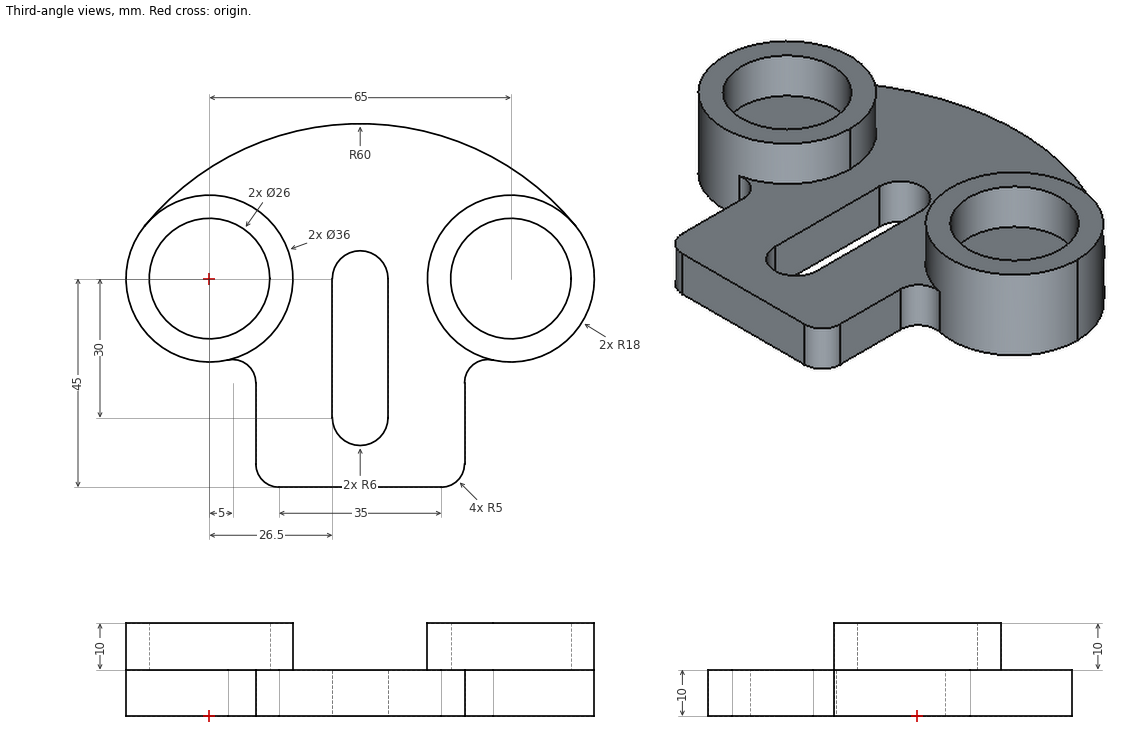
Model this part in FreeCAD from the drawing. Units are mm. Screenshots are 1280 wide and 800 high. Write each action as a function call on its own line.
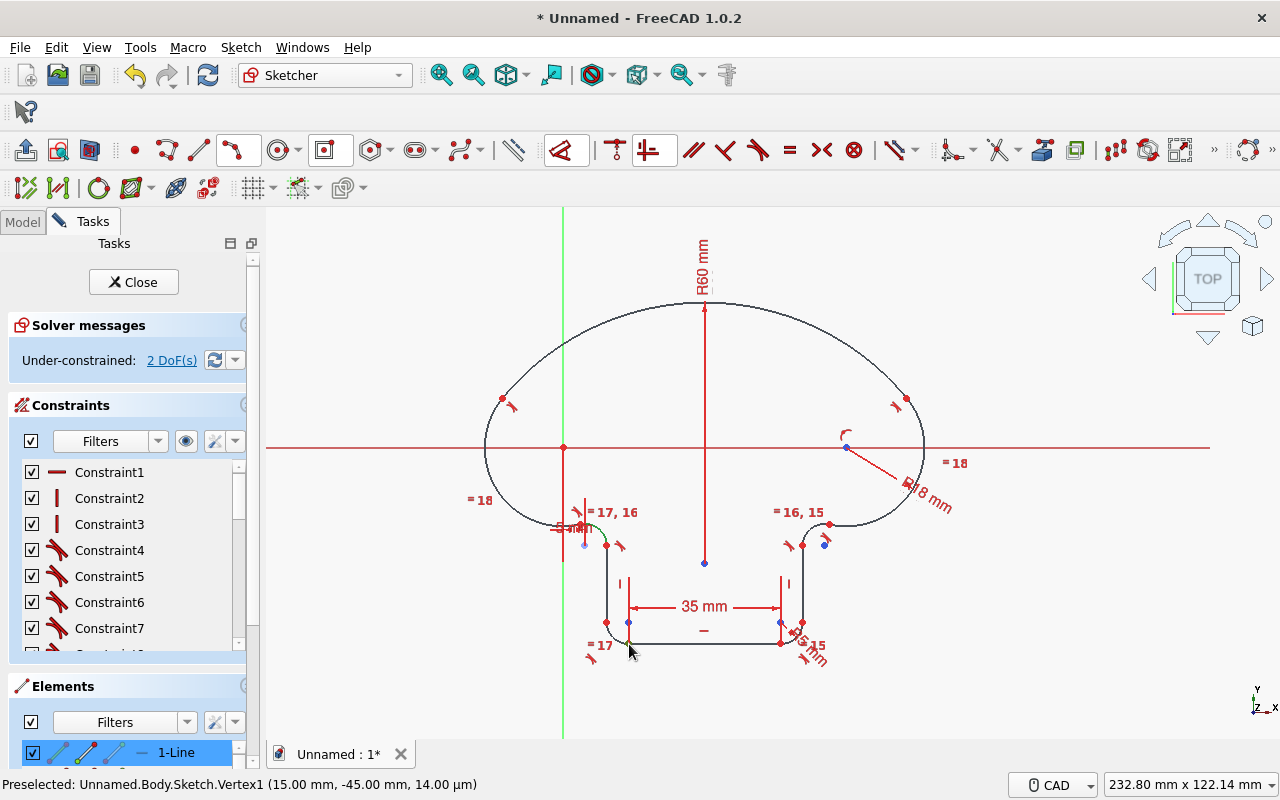
key(i)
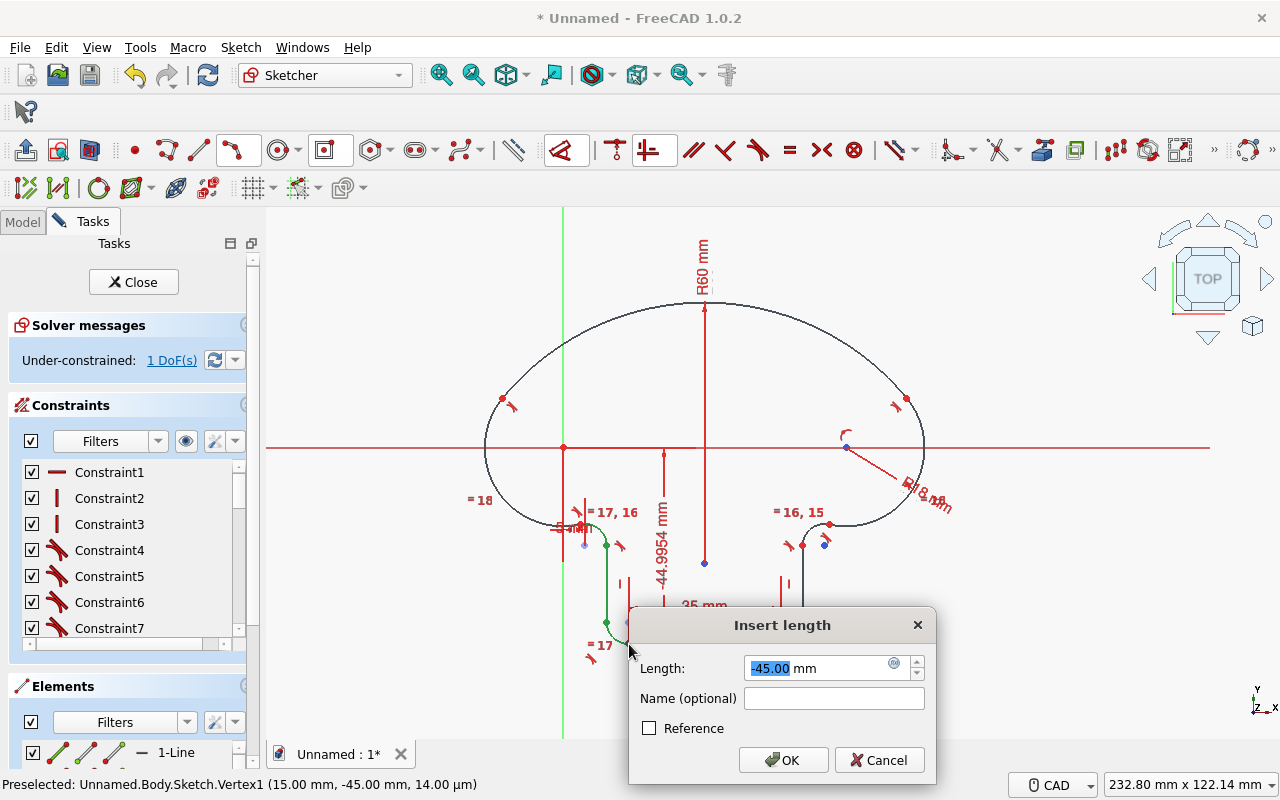
text(-45)
key(Return)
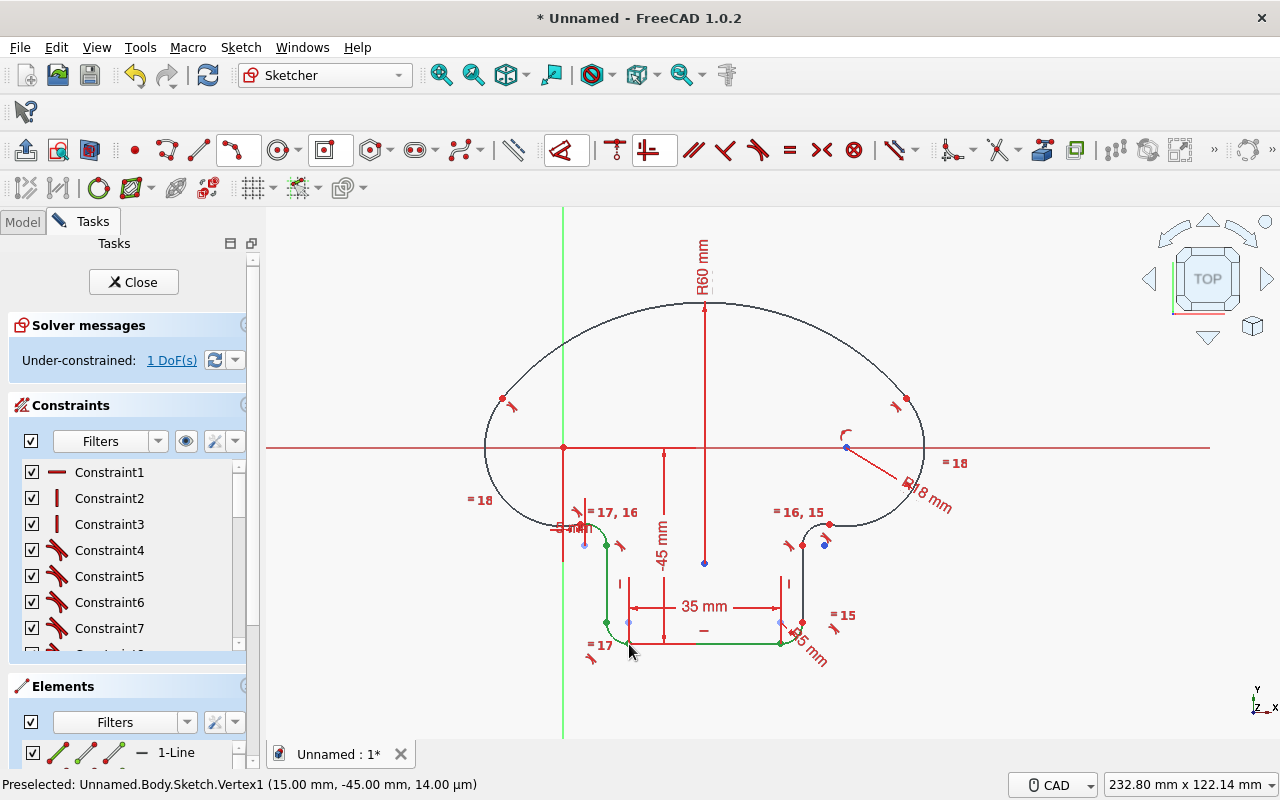
click(846, 448)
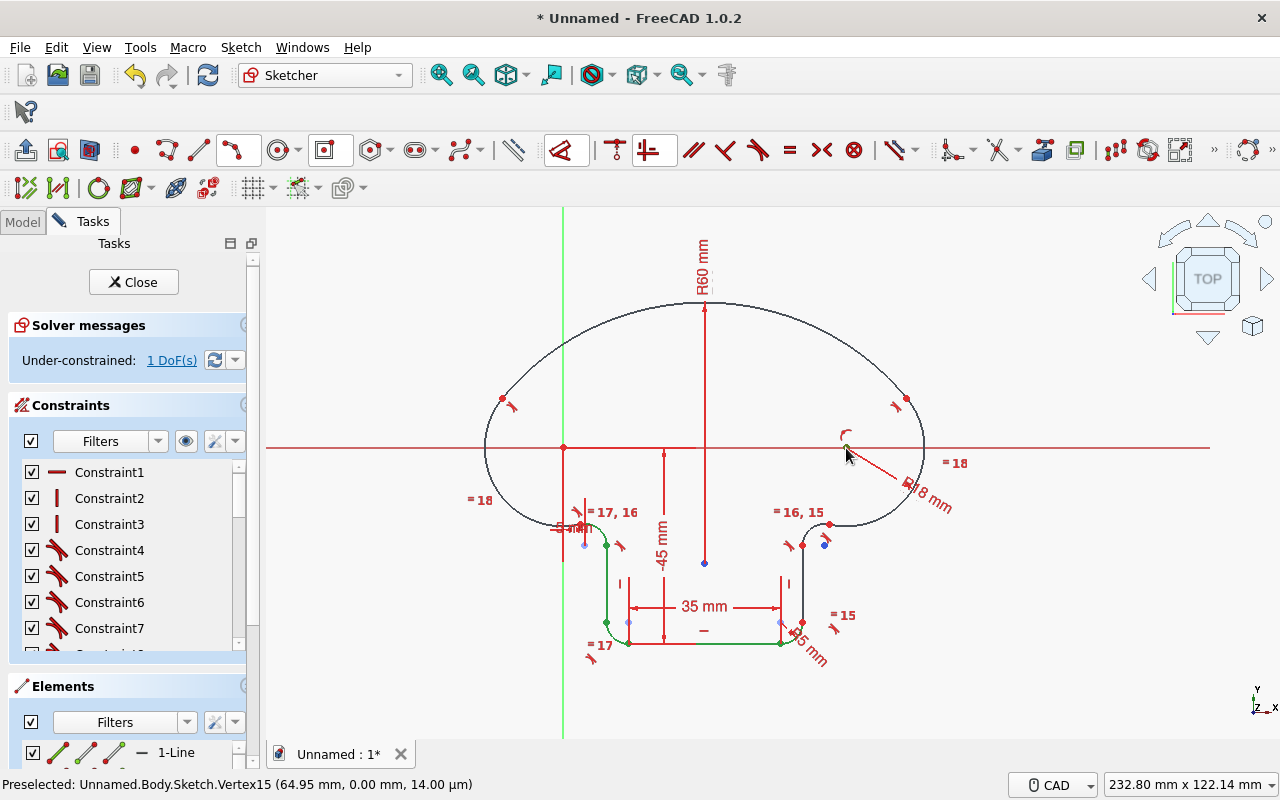
click(584, 150)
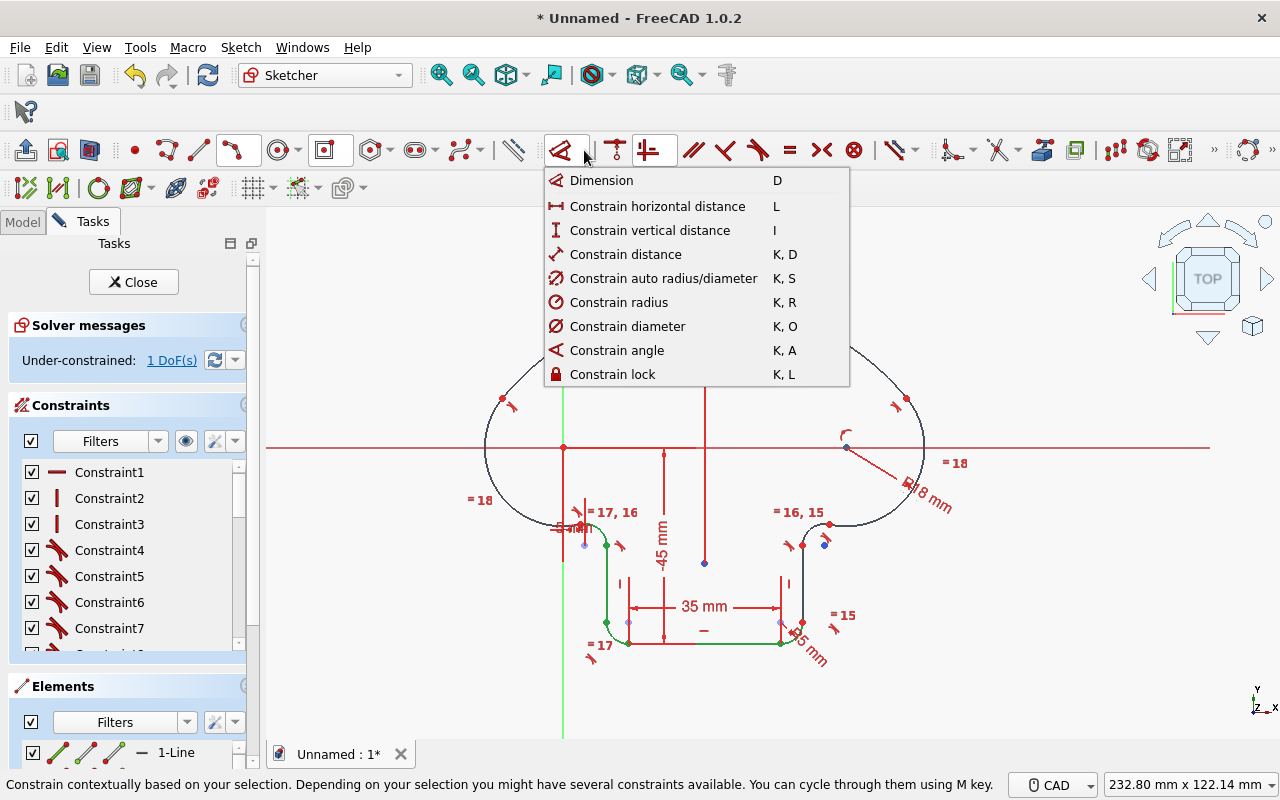
click(697, 206)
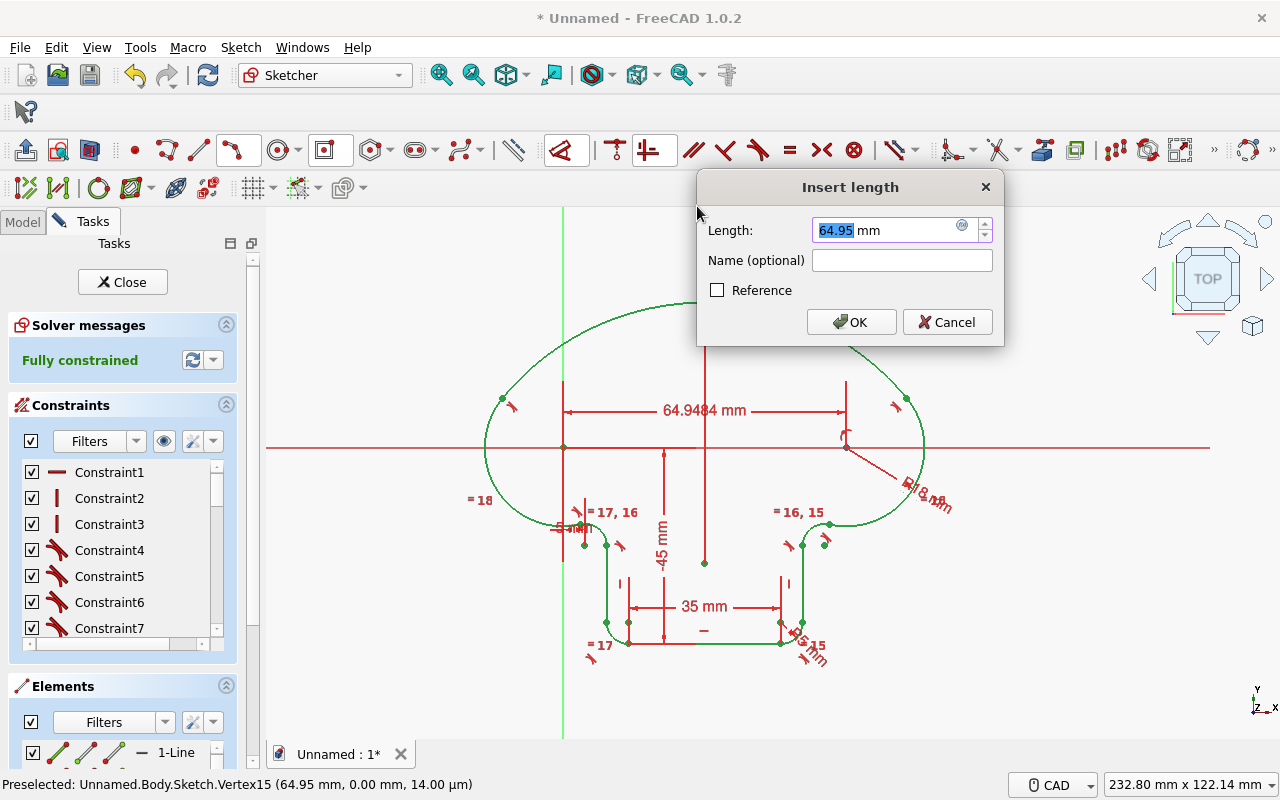
text(65)
key(Return)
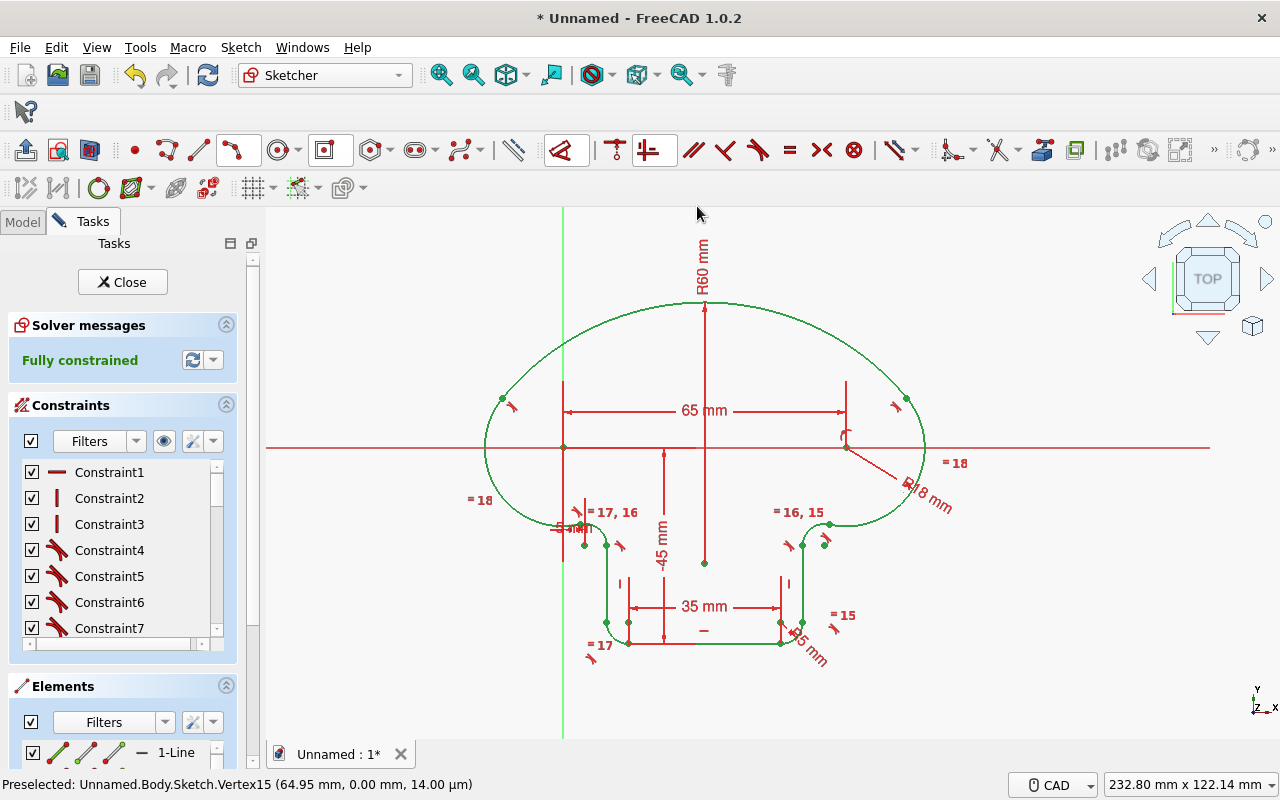
click(123, 282)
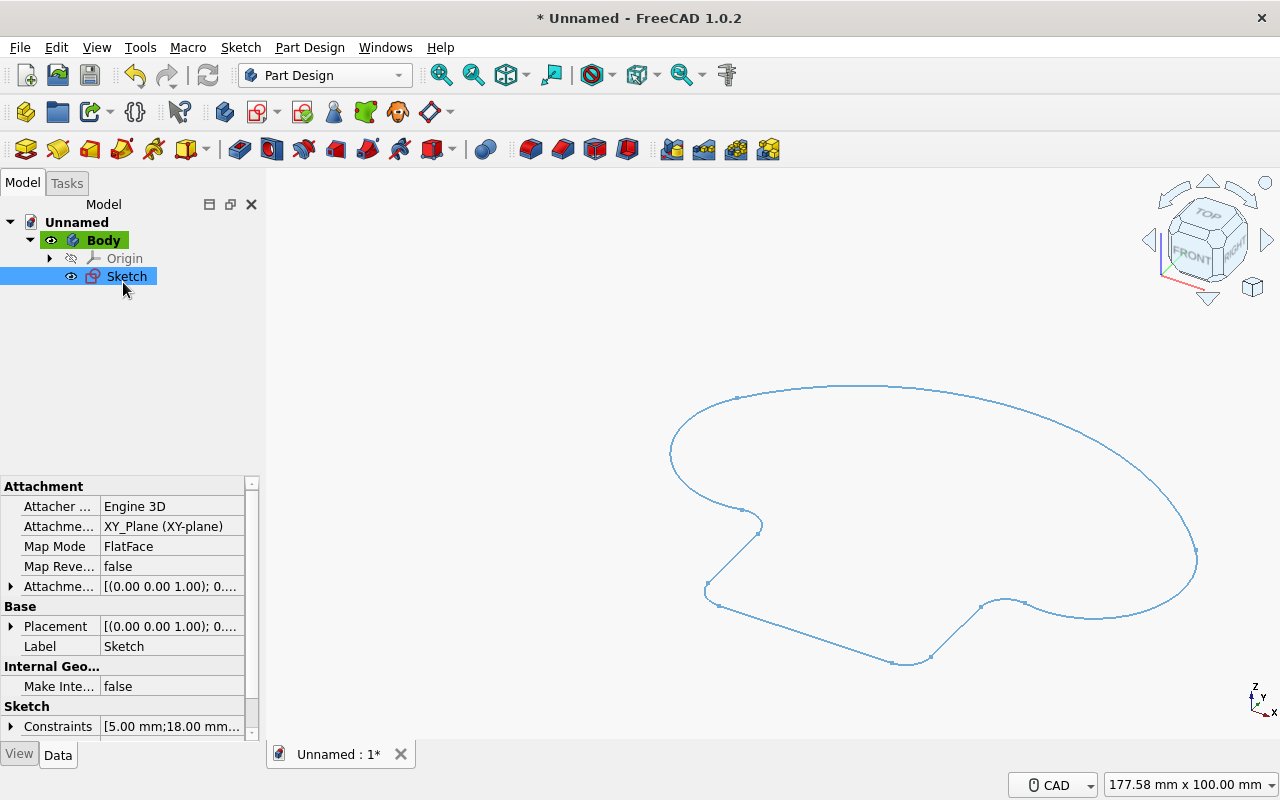
click(26, 150)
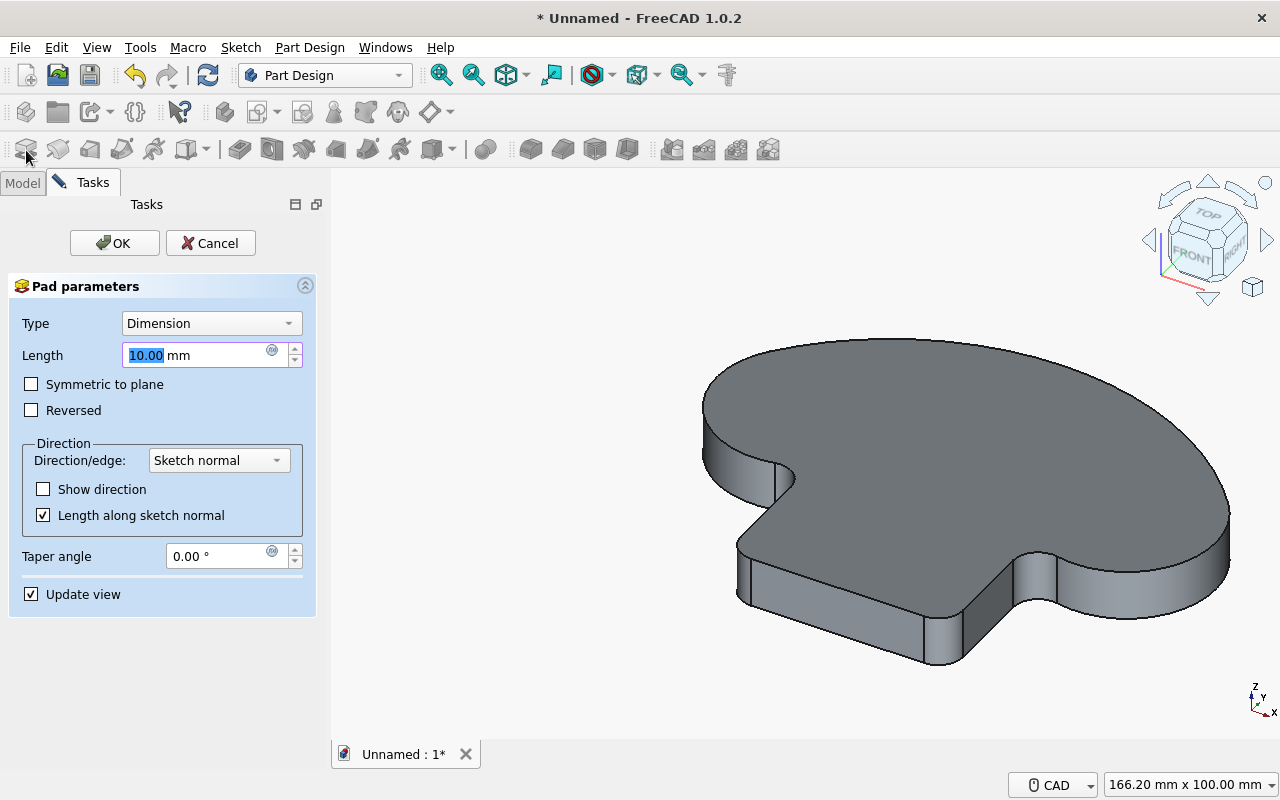
text(10)
key(Tab)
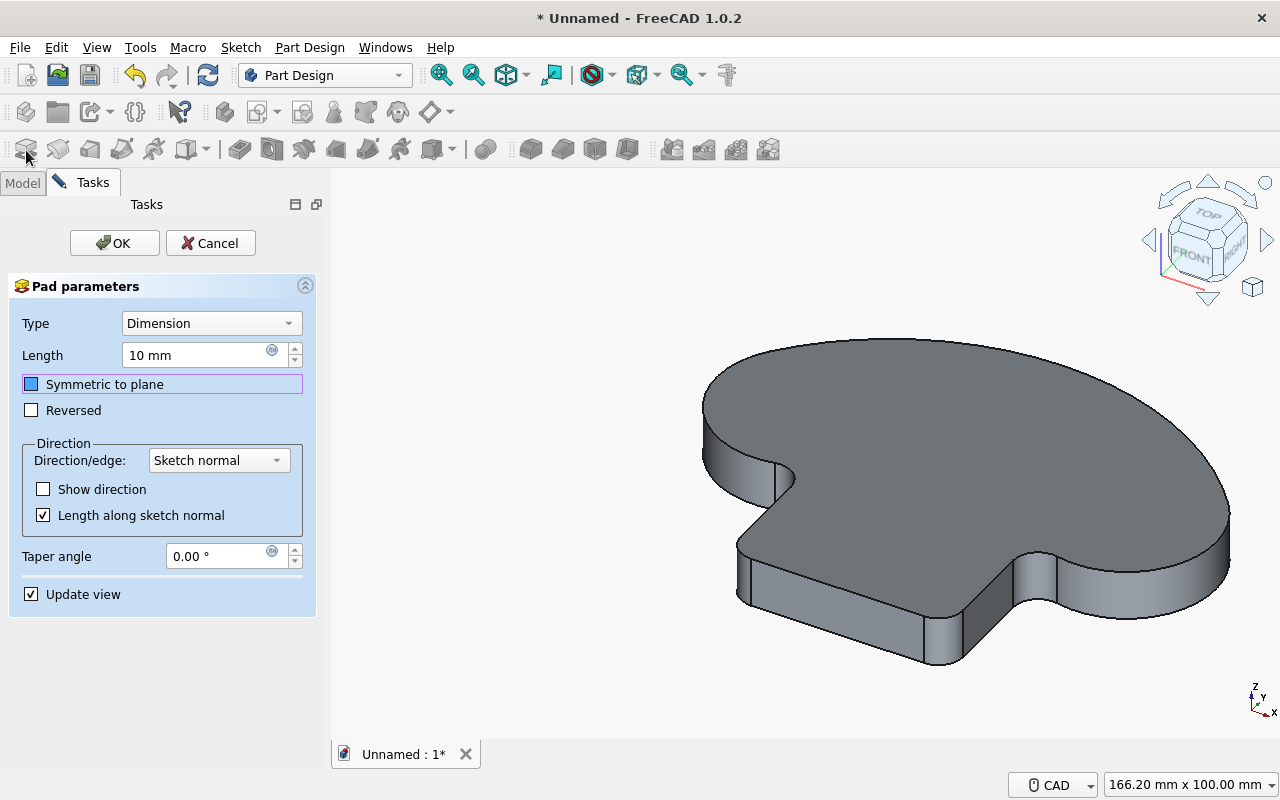
click(115, 243)